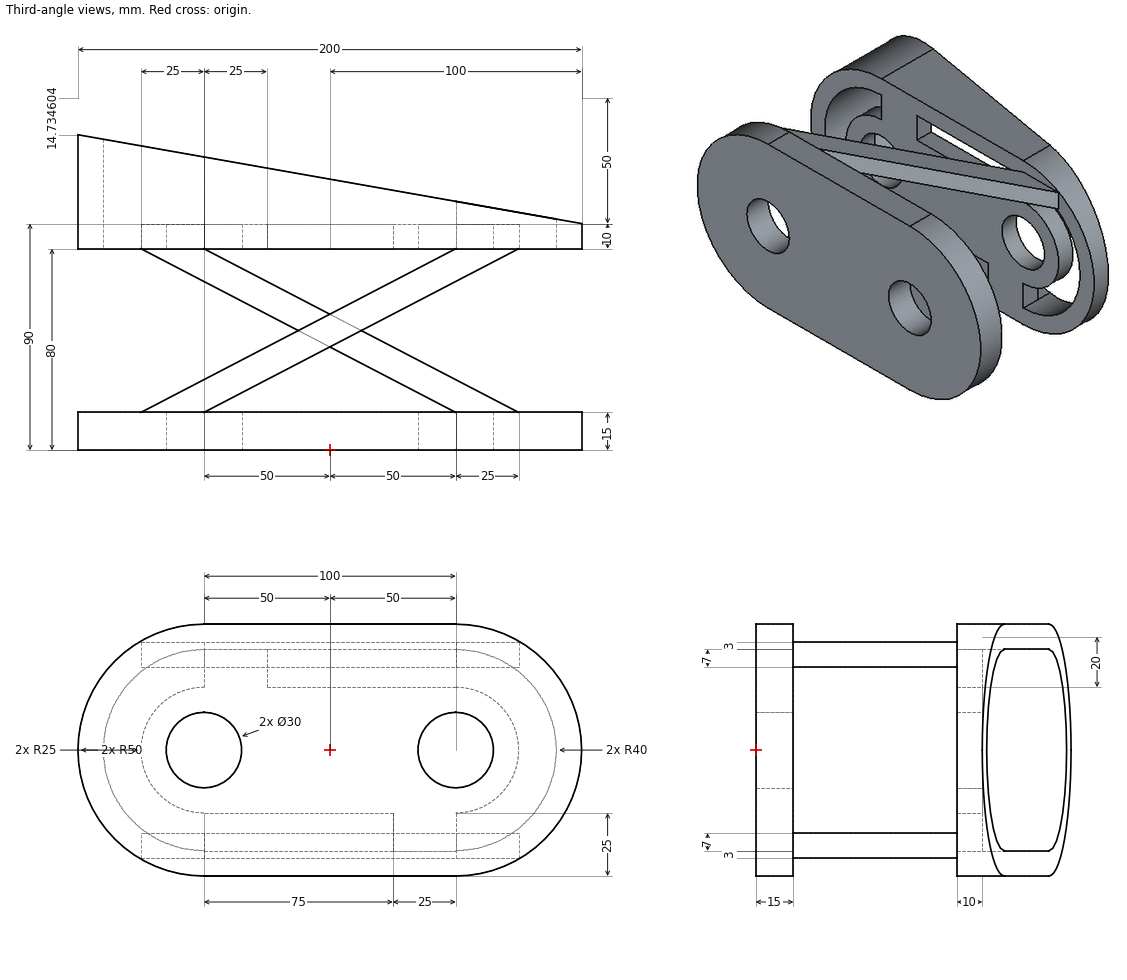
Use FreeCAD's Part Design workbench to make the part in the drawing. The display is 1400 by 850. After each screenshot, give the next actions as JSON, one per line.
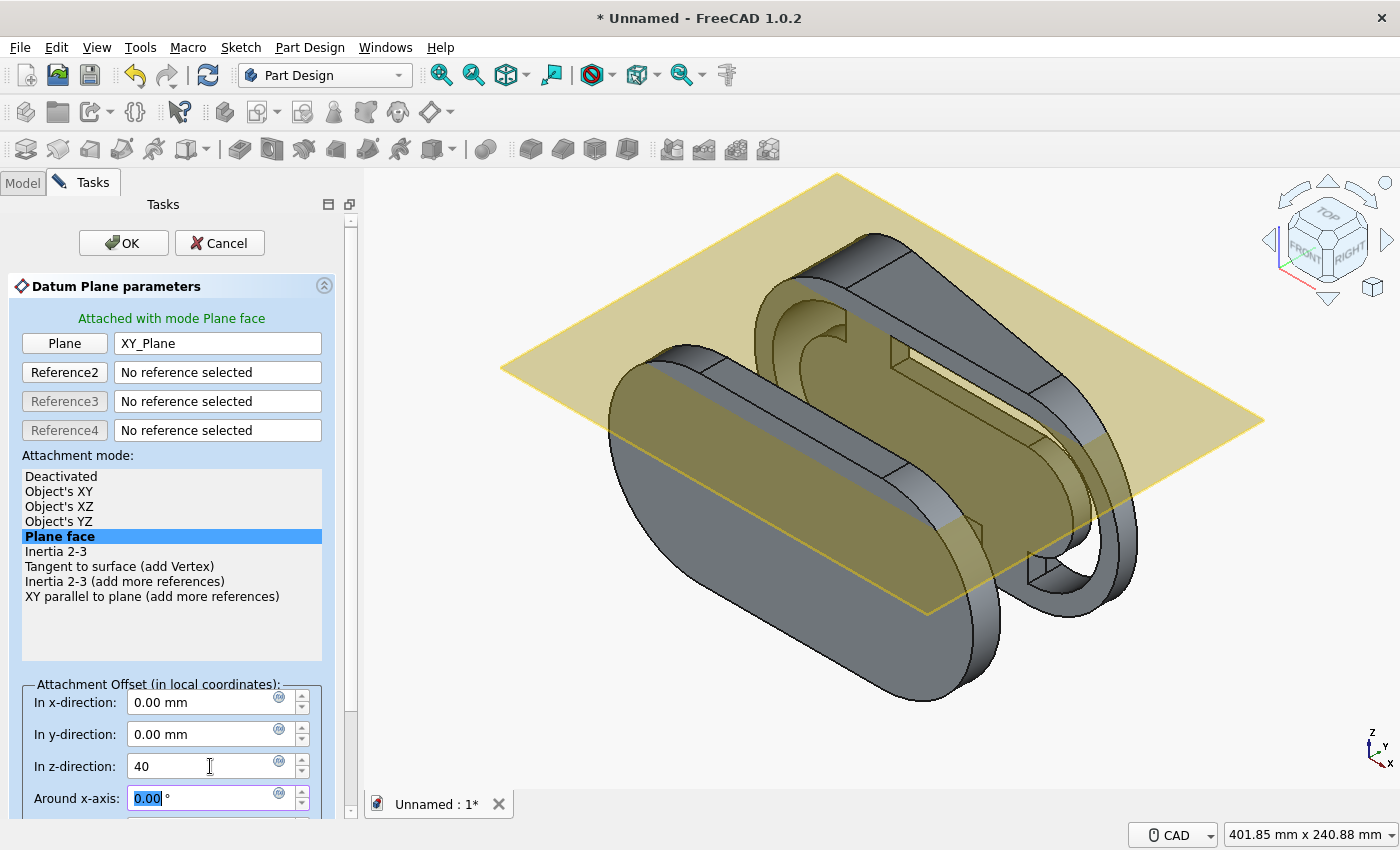
{"action": "left_click", "coordinate": [124, 243]}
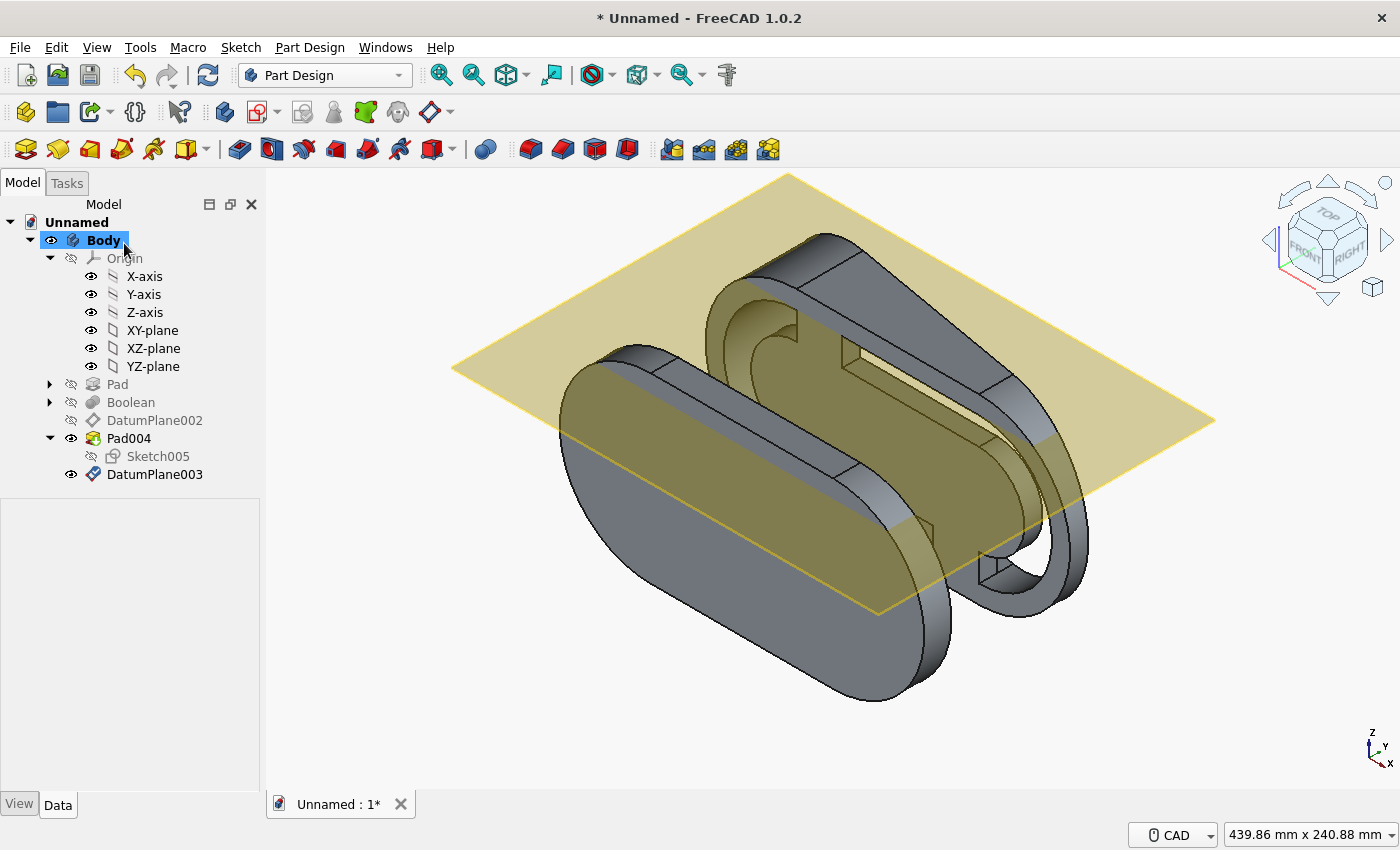
{"action": "left_click", "coordinate": [116, 474]}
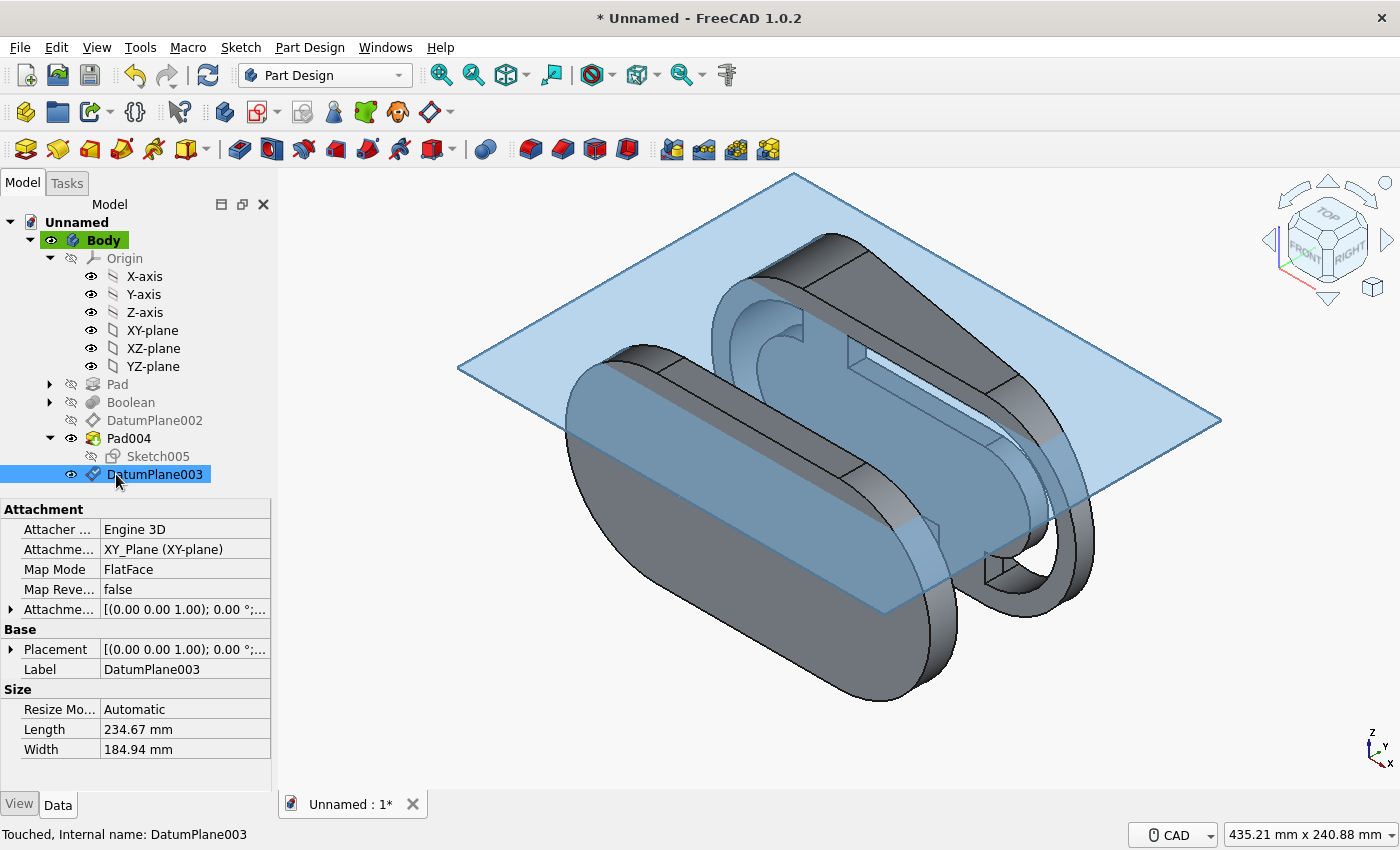
{"action": "left_click", "coordinate": [258, 112]}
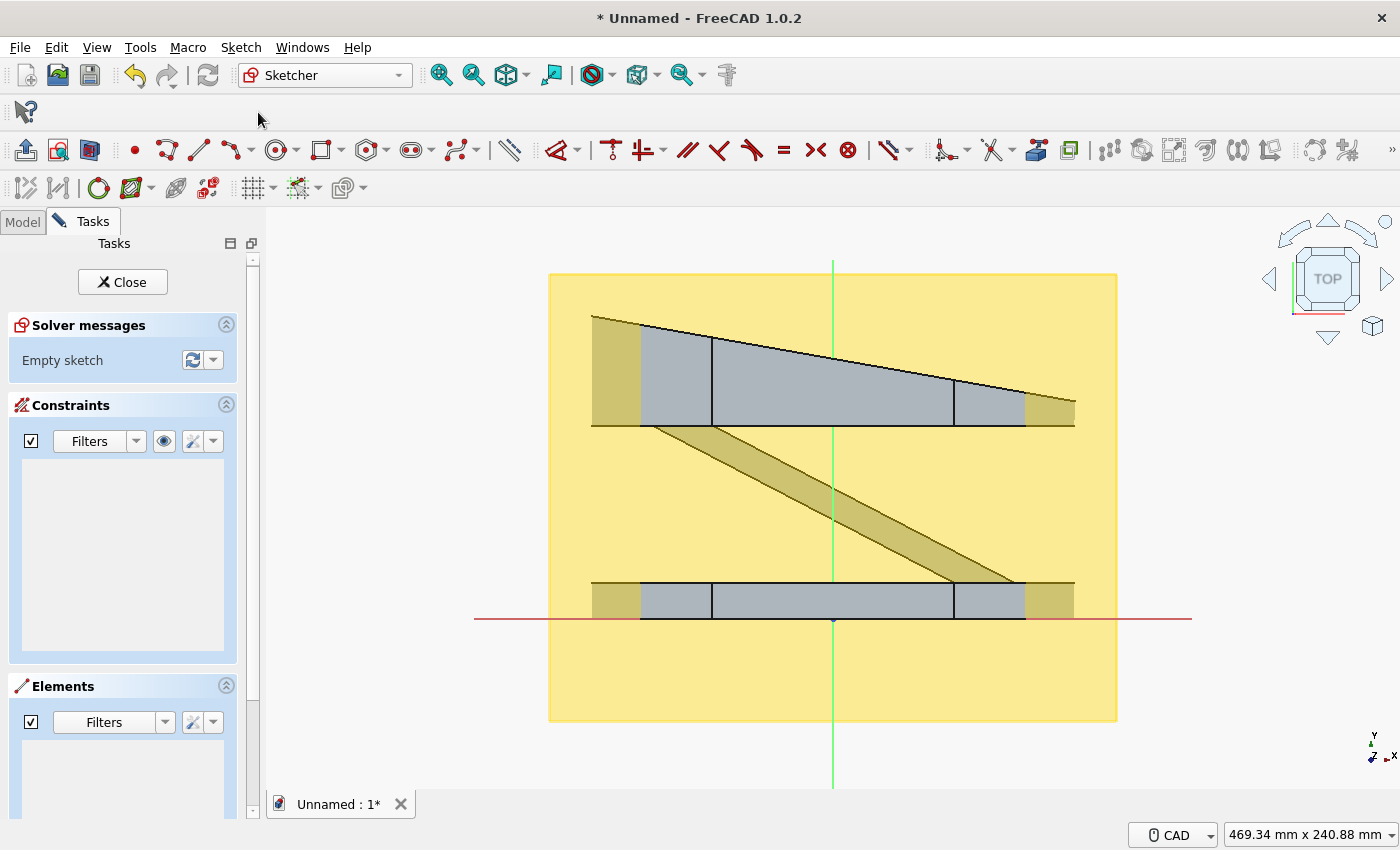
{"action": "left_click", "coordinate": [90, 150]}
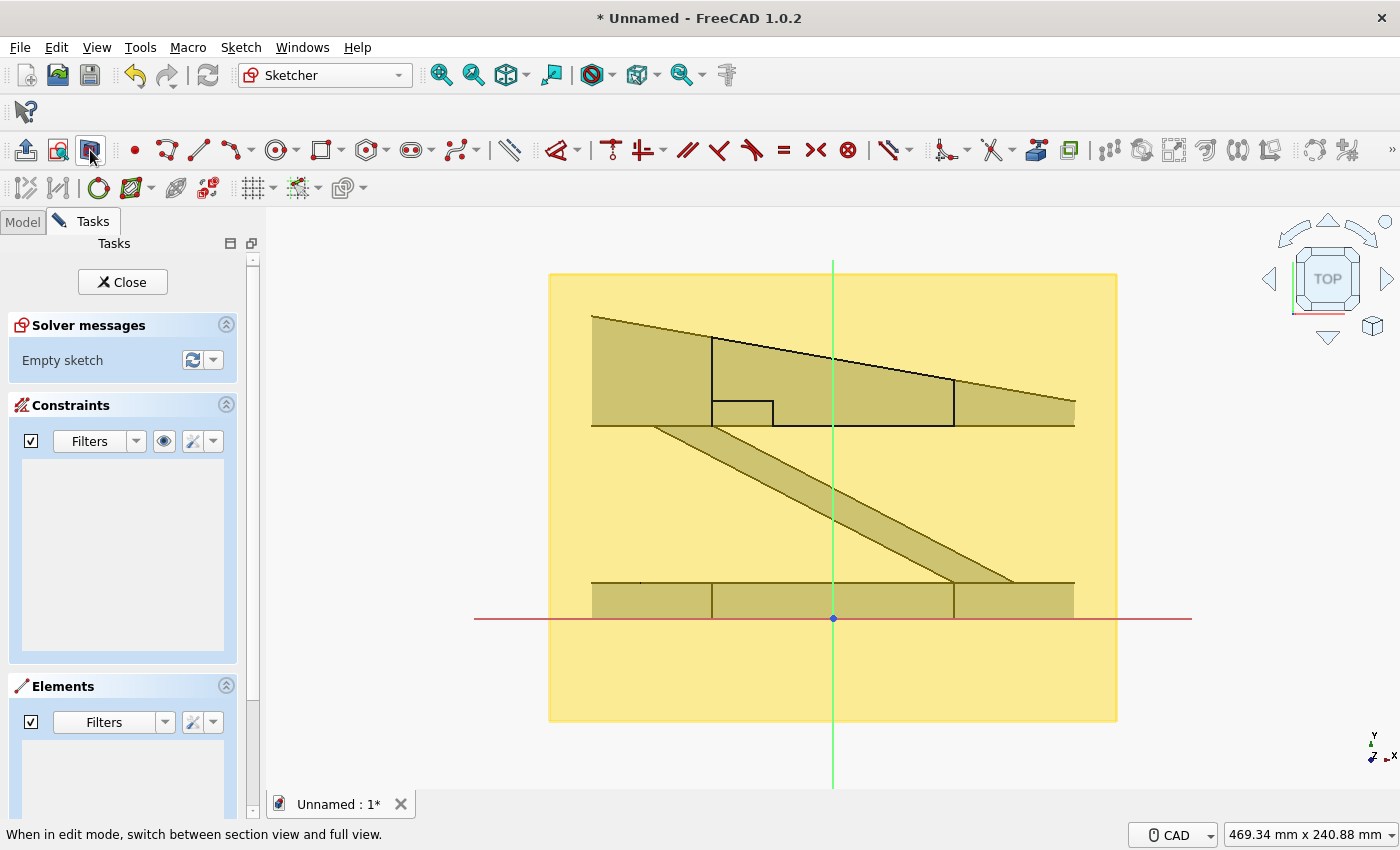
{"action": "scroll", "coordinate": [917, 552], "scroll_direction": "up", "scroll_amount": 3}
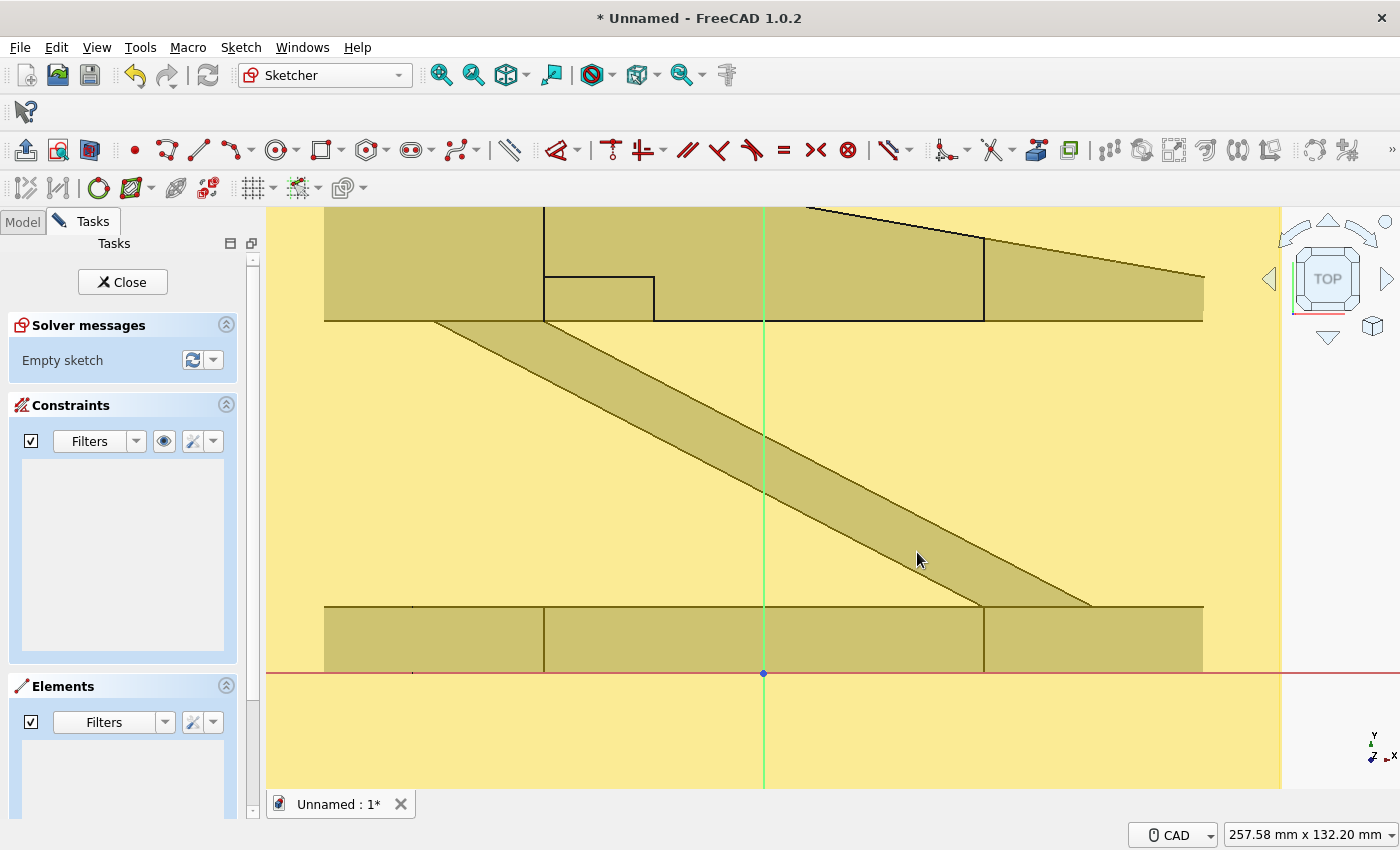
{"action": "left_click", "coordinate": [168, 150]}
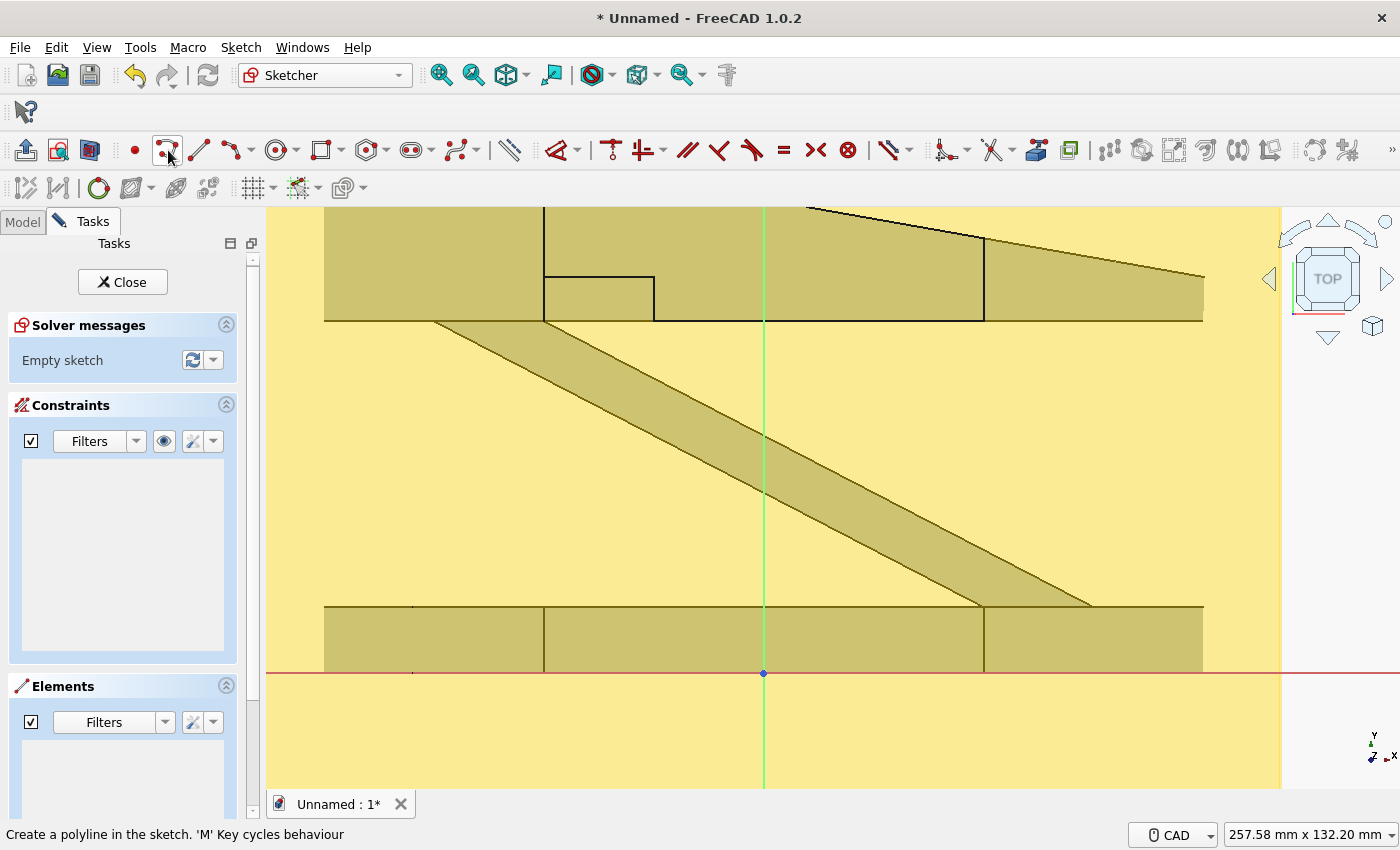
{"action": "left_click", "coordinate": [544, 607]}
{"action": "left_click", "coordinate": [434, 607]}
{"action": "left_click", "coordinate": [984, 321]}
{"action": "left_click", "coordinate": [1094, 321]}
{"action": "left_click", "coordinate": [544, 608]}
{"action": "key", "text": "Escape"}
{"action": "key", "text": "Escape"}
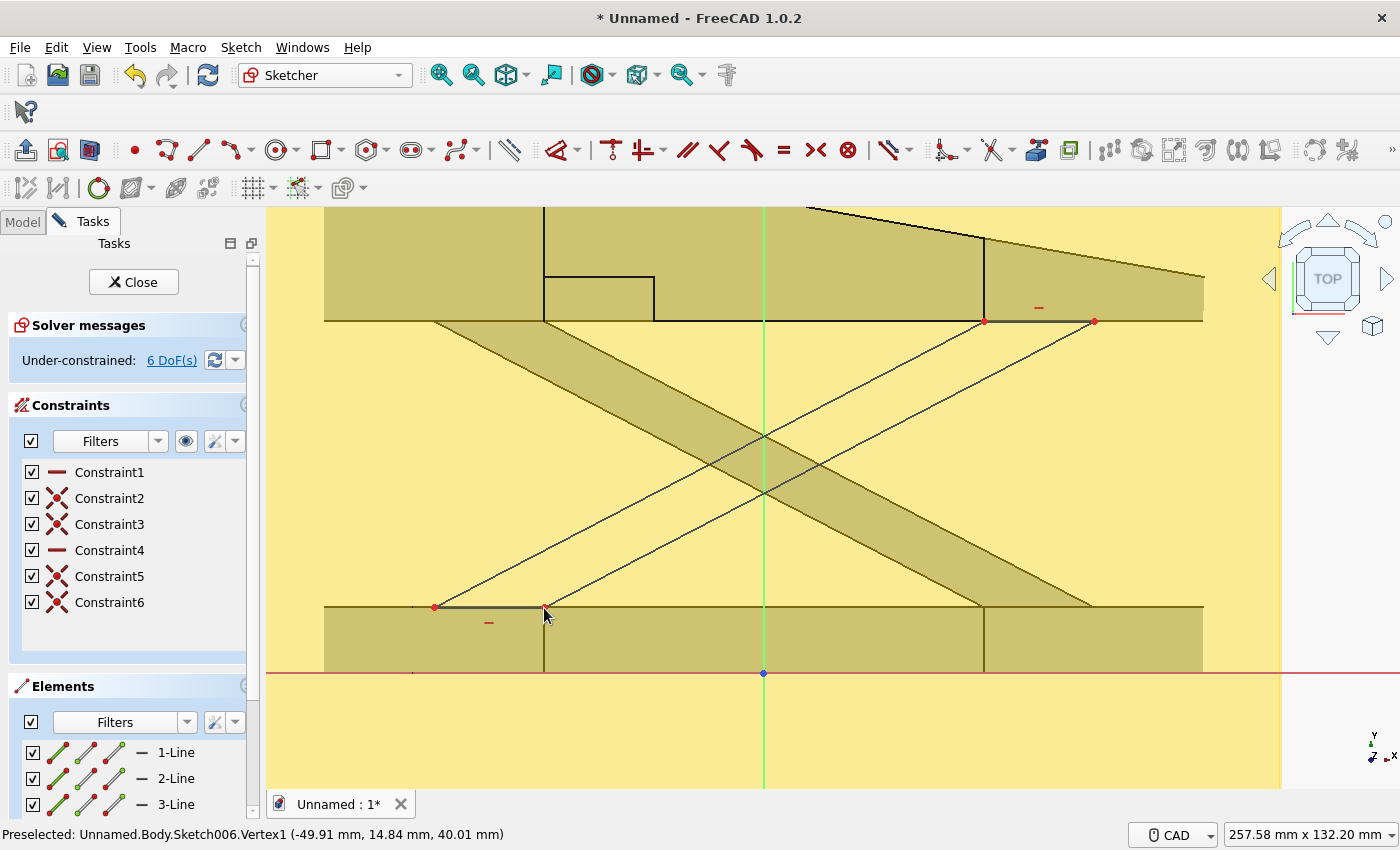
{"action": "left_click", "coordinate": [556, 150]}